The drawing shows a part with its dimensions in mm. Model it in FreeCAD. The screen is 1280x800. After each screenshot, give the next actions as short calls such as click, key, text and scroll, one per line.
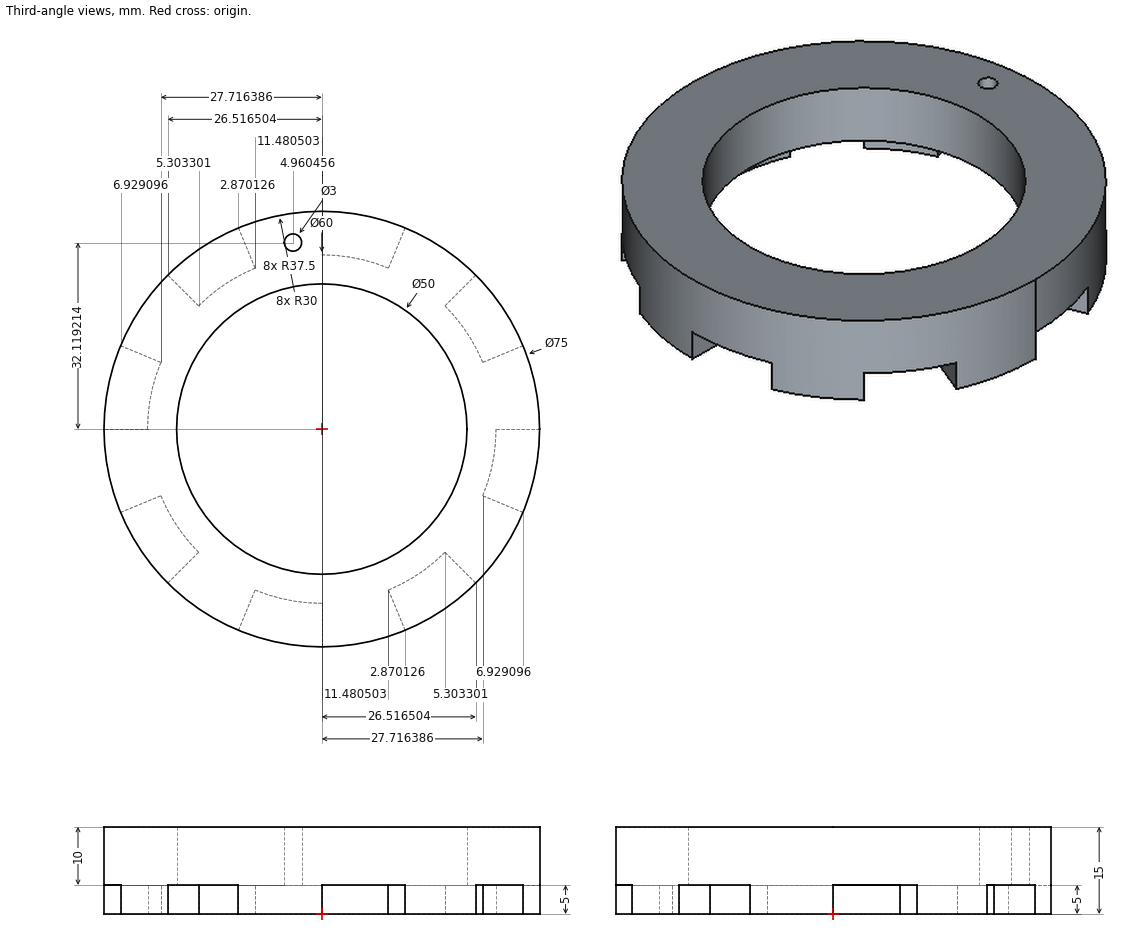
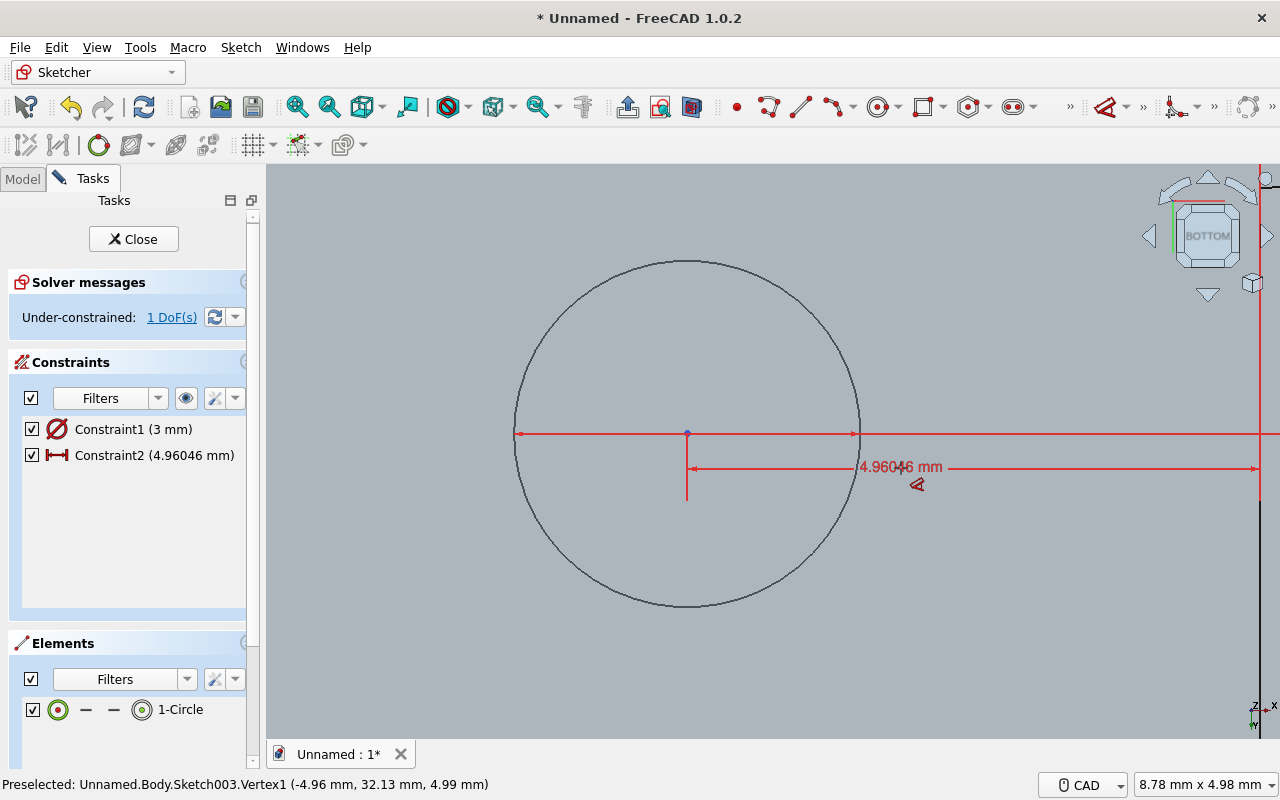
click(687, 434)
click(653, 313)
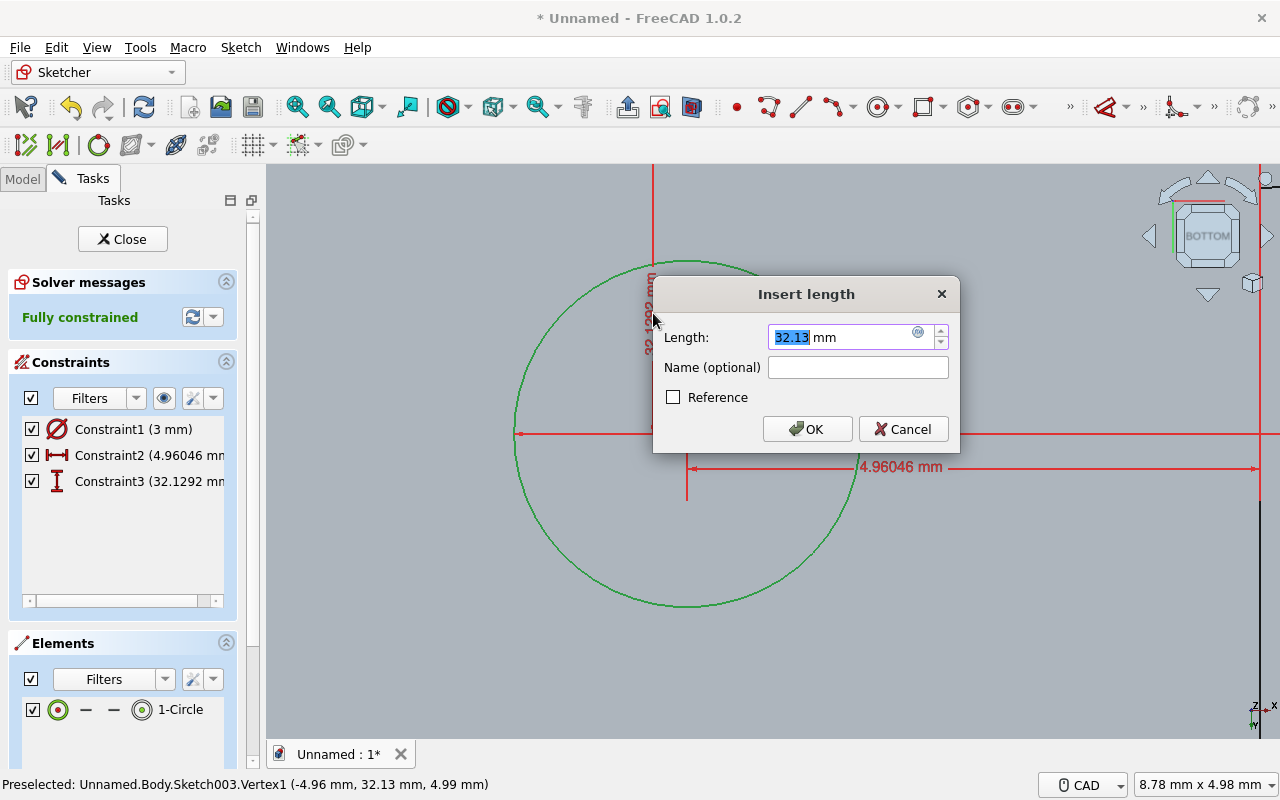
text(32.119214)
key(Return)
key(Escape)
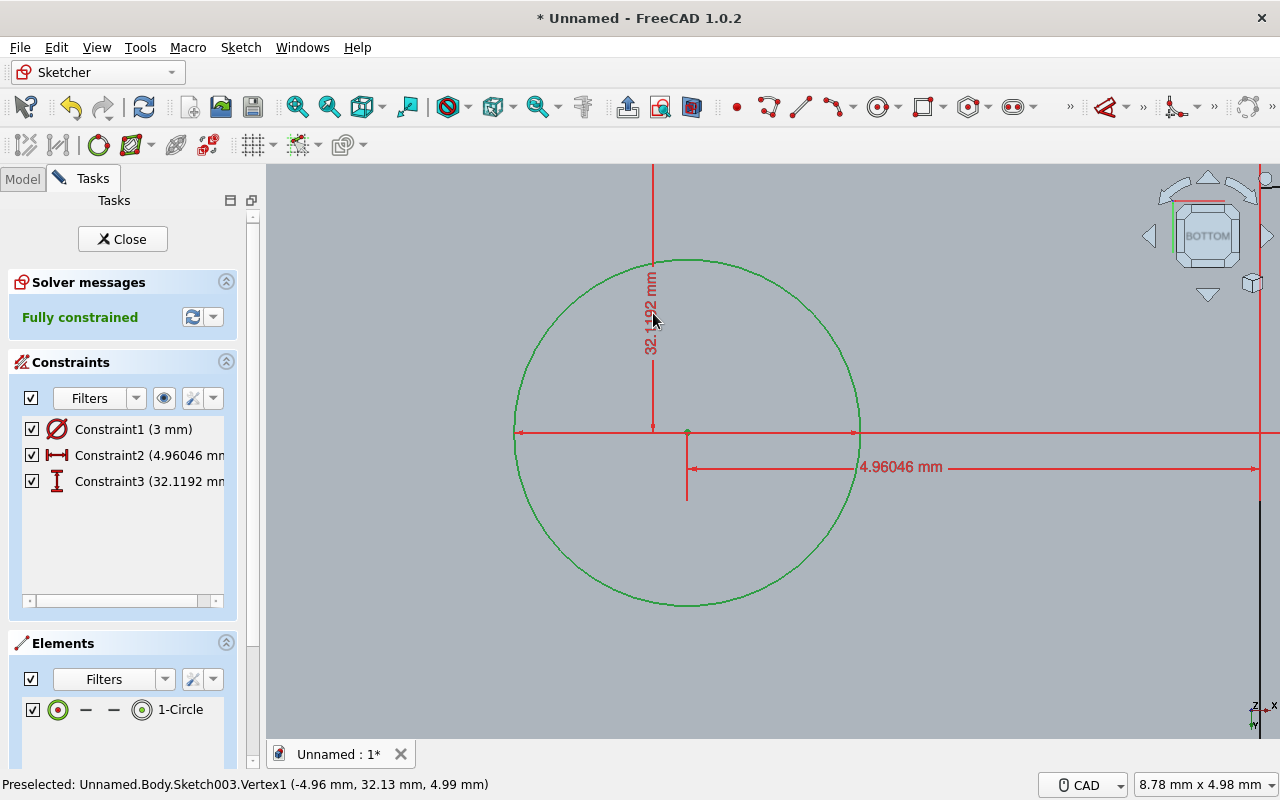
click(123, 239)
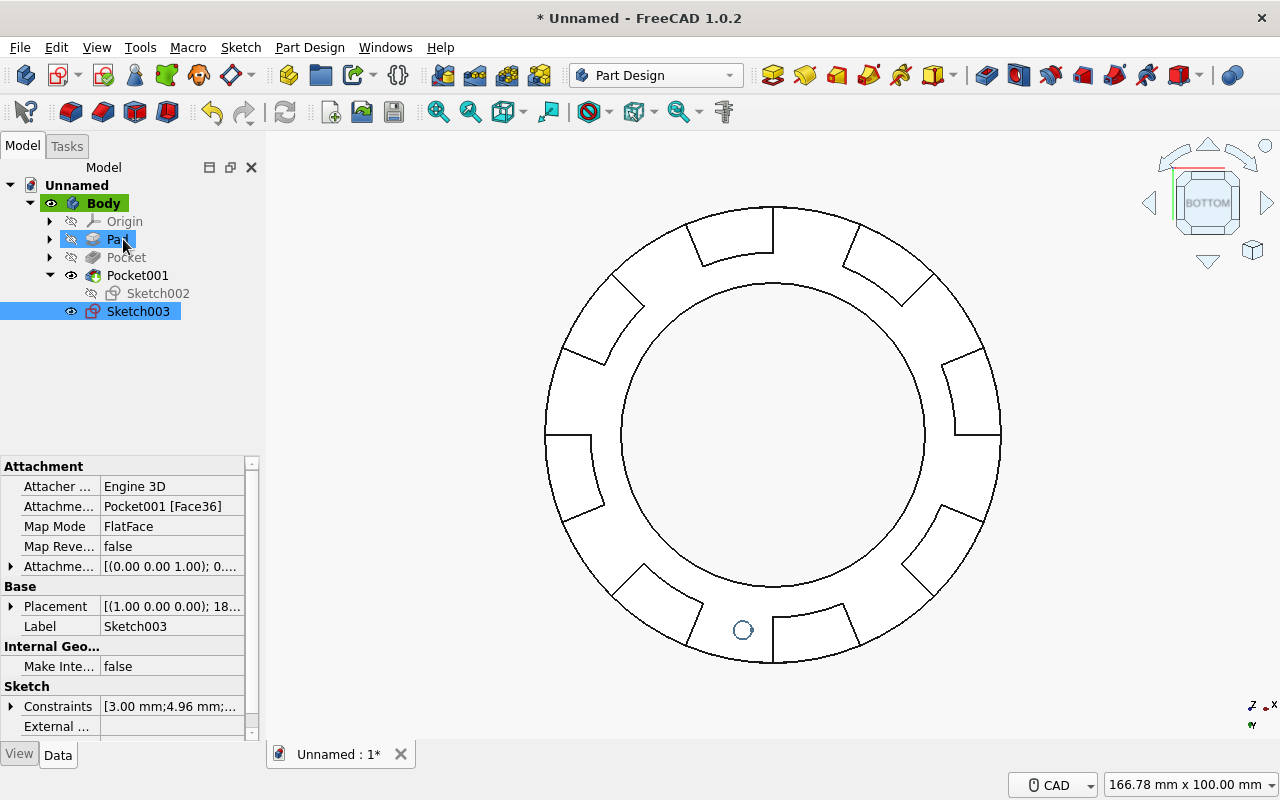
click(988, 76)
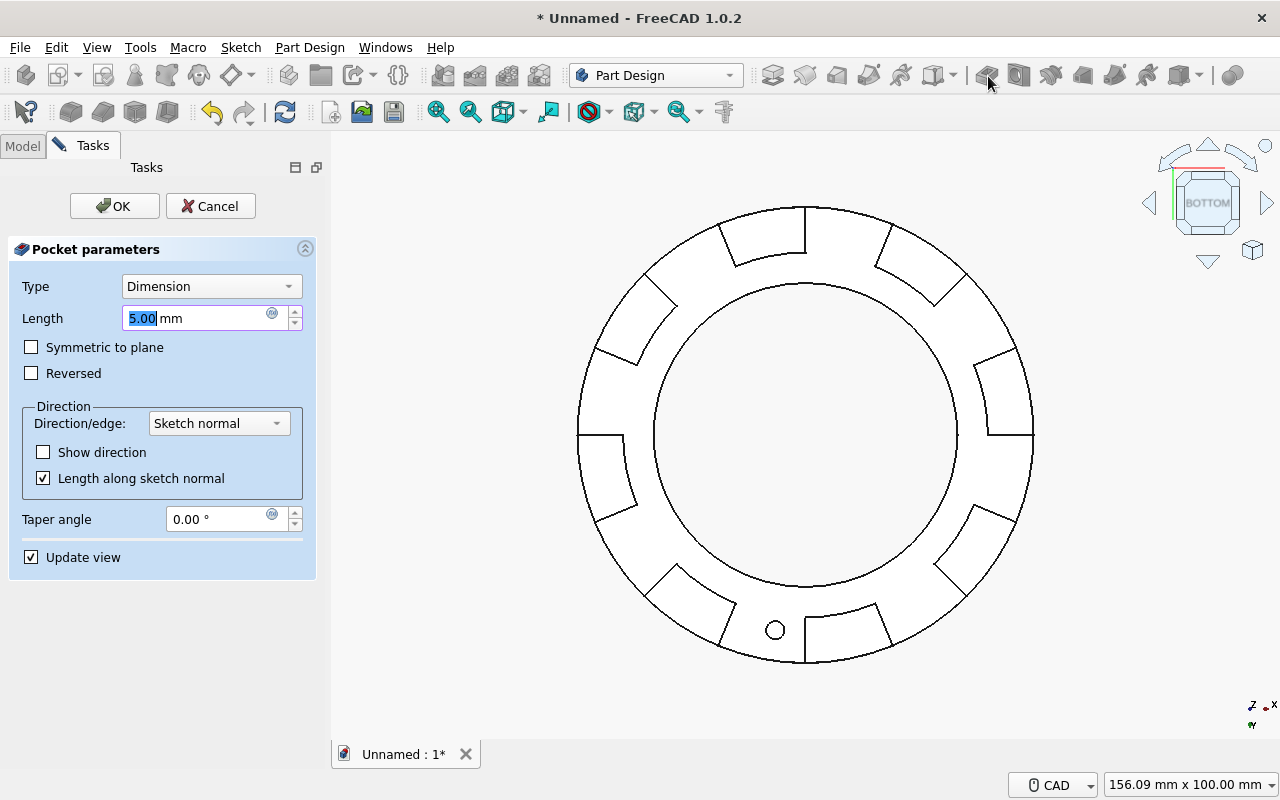
text(10)
key(Tab)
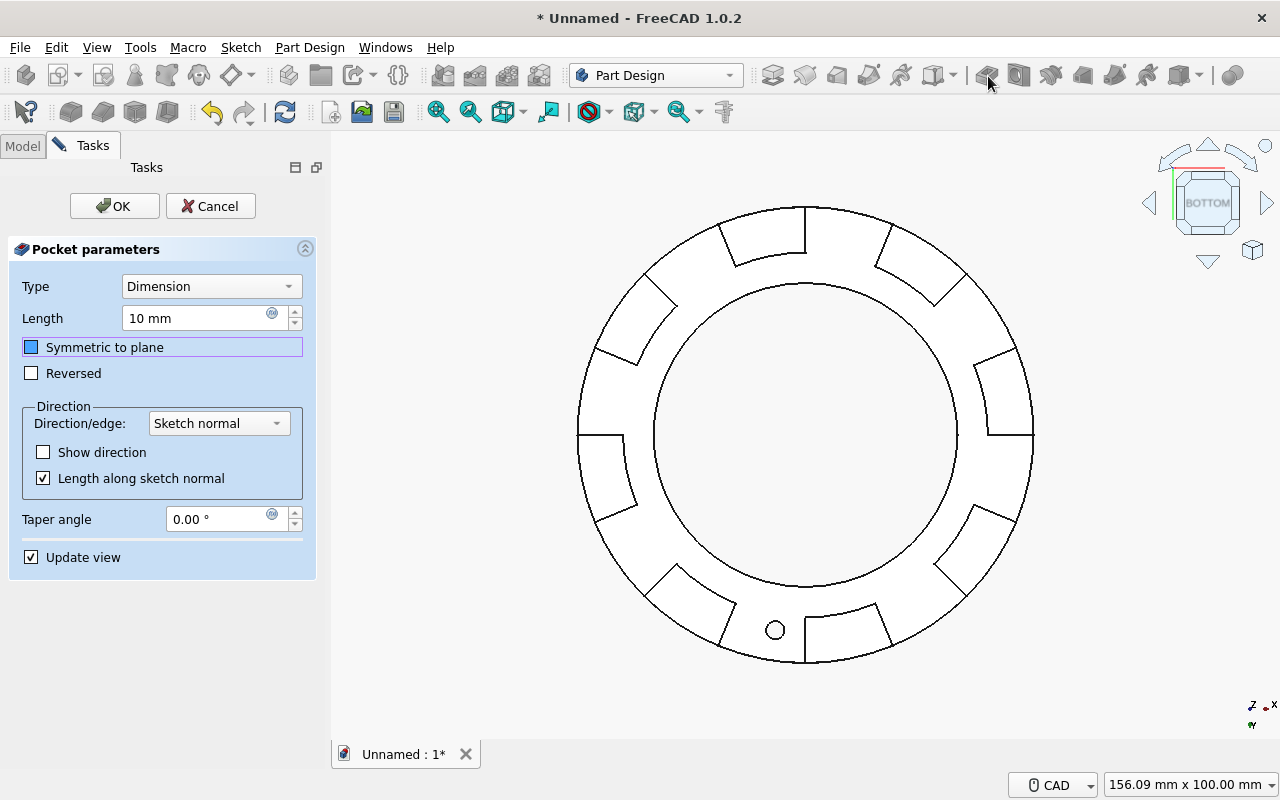
click(115, 206)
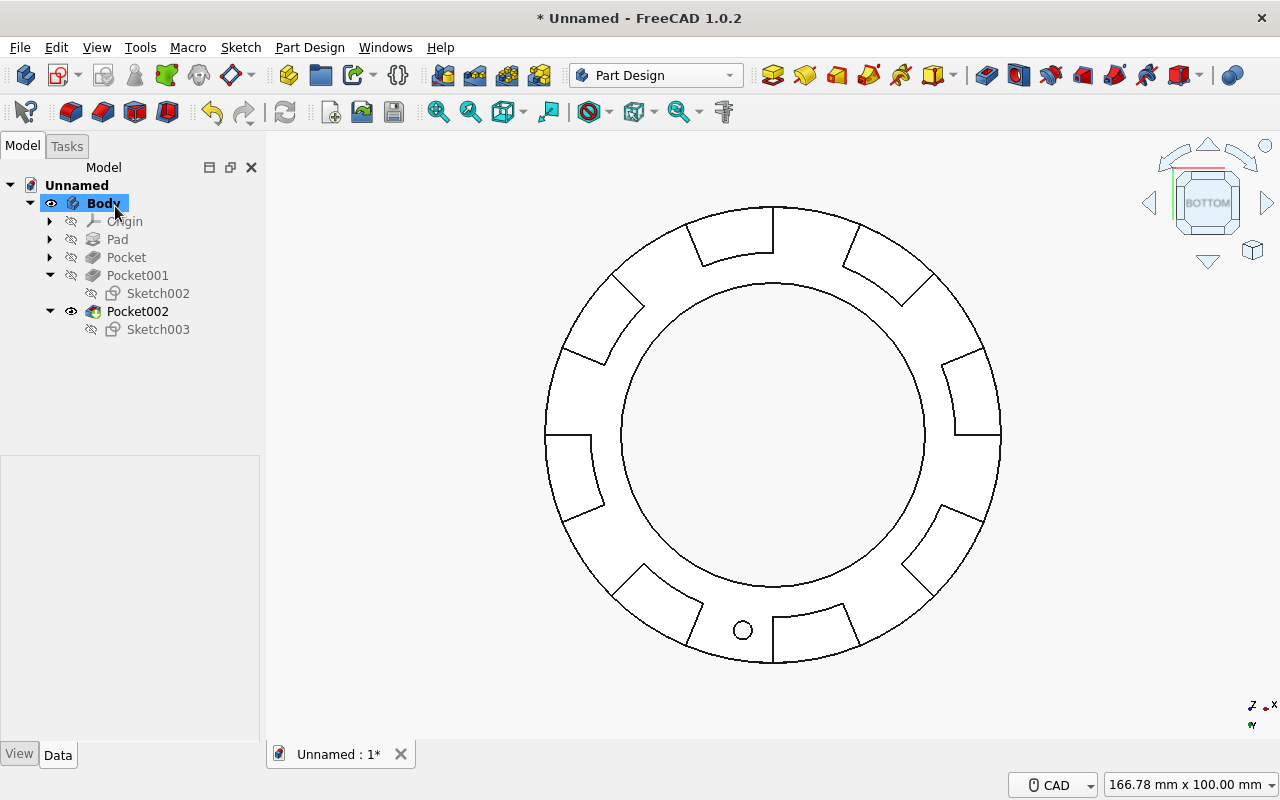
key(0)